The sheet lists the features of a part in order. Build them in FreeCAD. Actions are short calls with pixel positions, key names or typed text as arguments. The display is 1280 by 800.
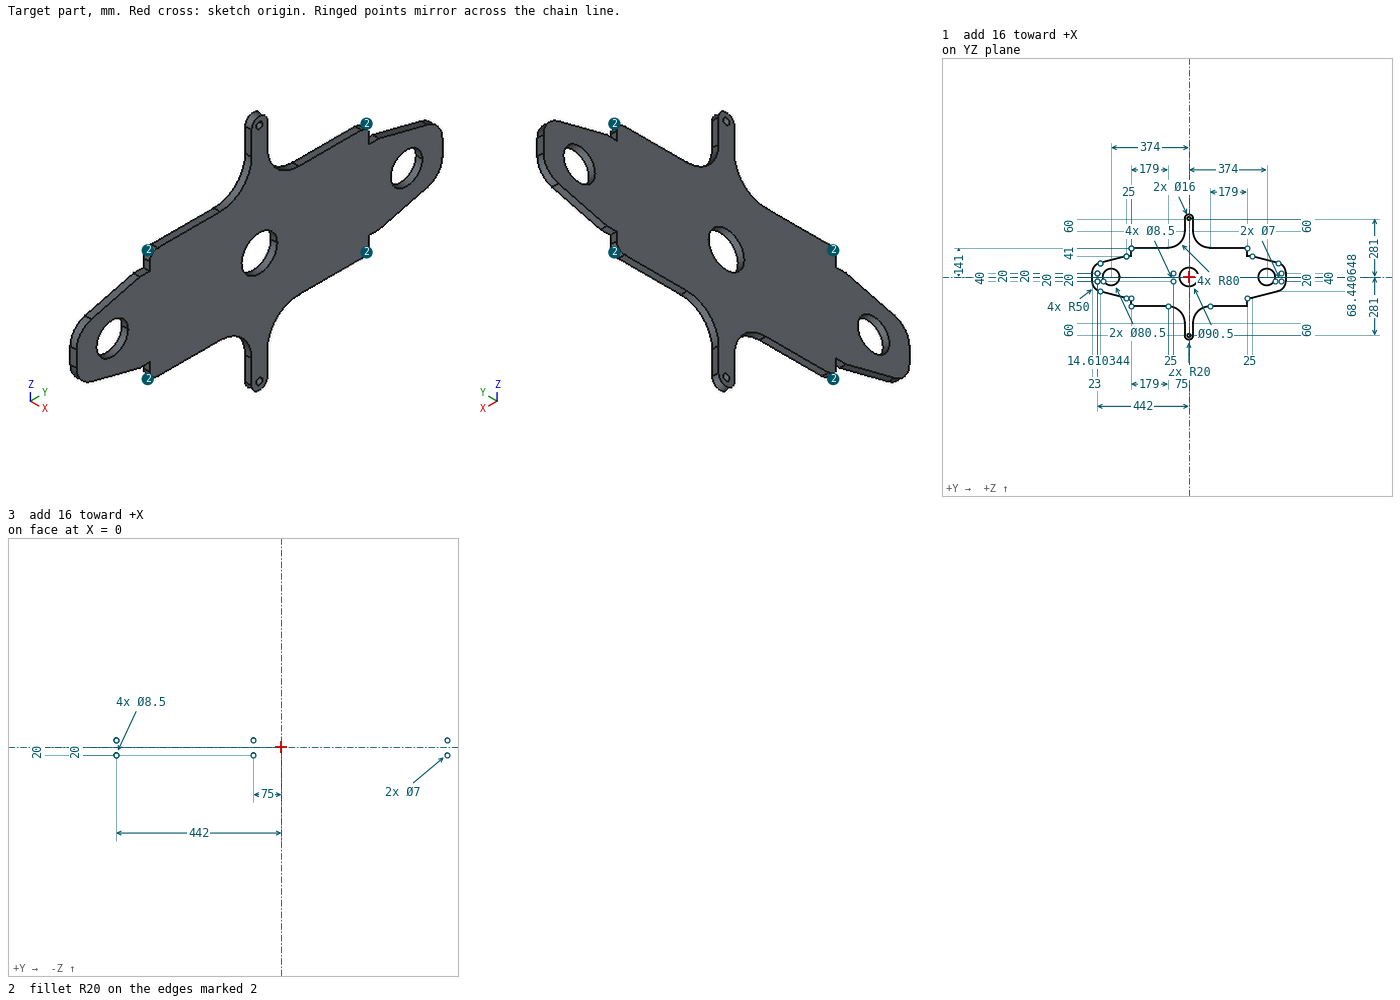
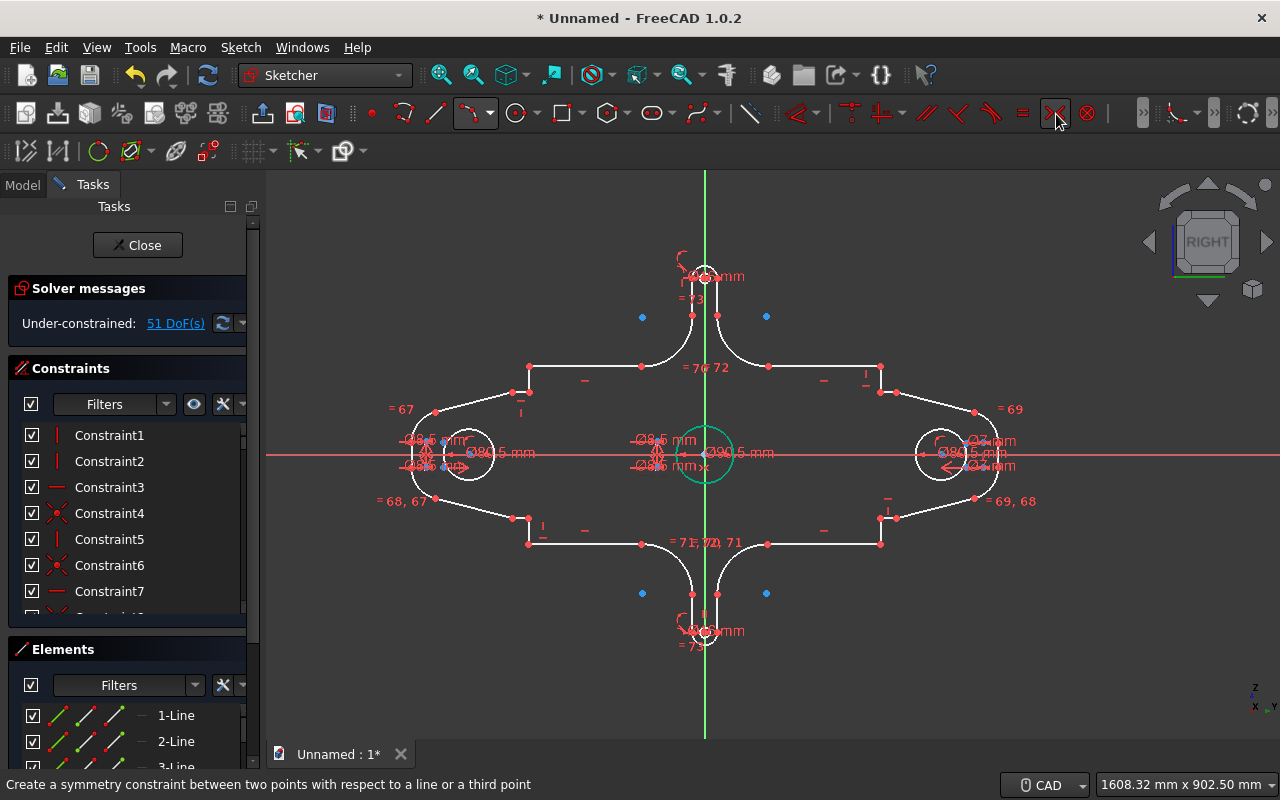
click(426, 468)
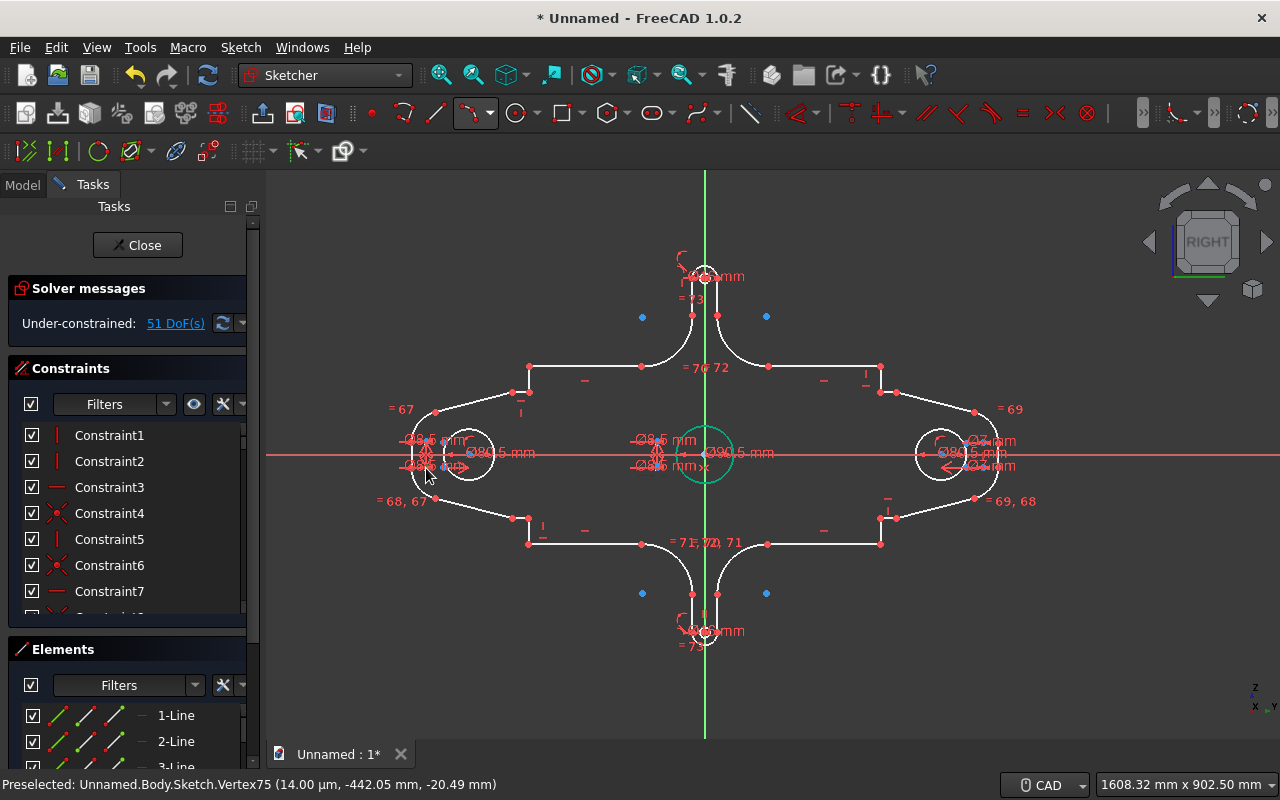
click(983, 468)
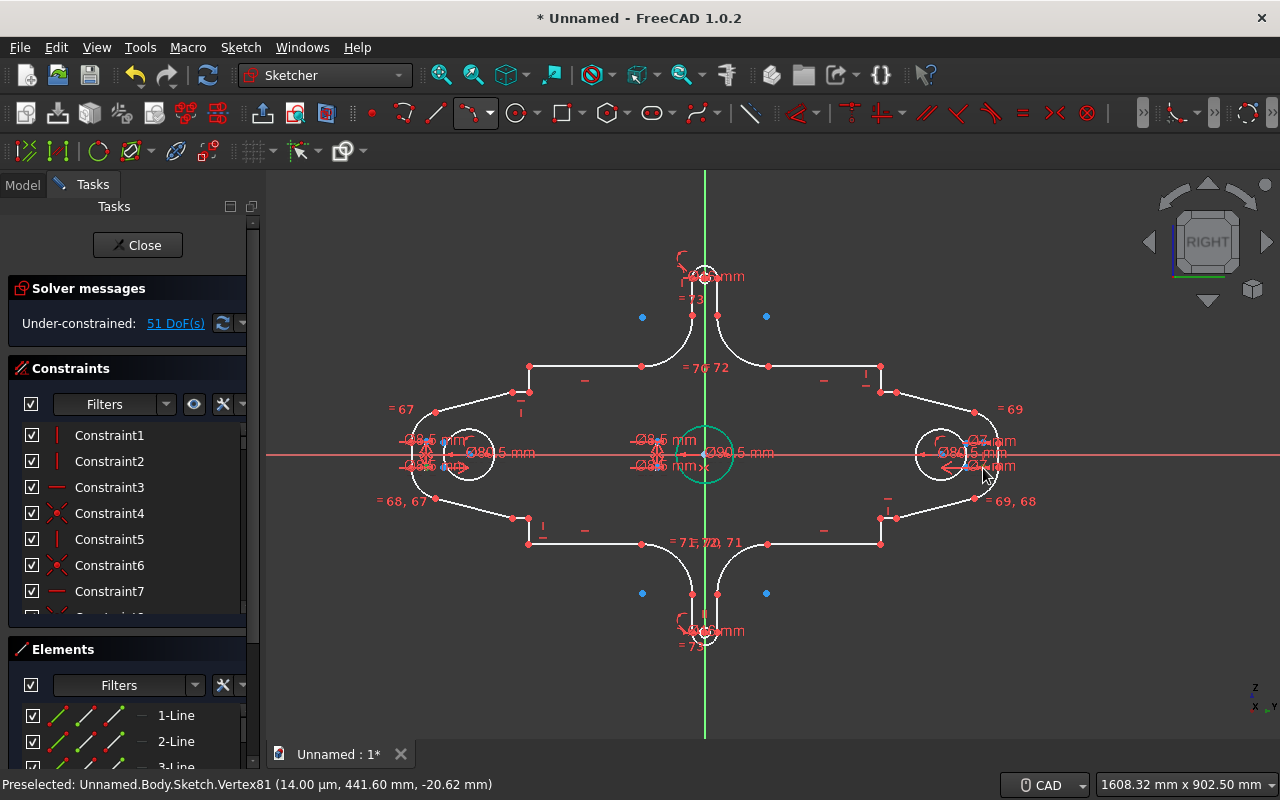
click(705, 528)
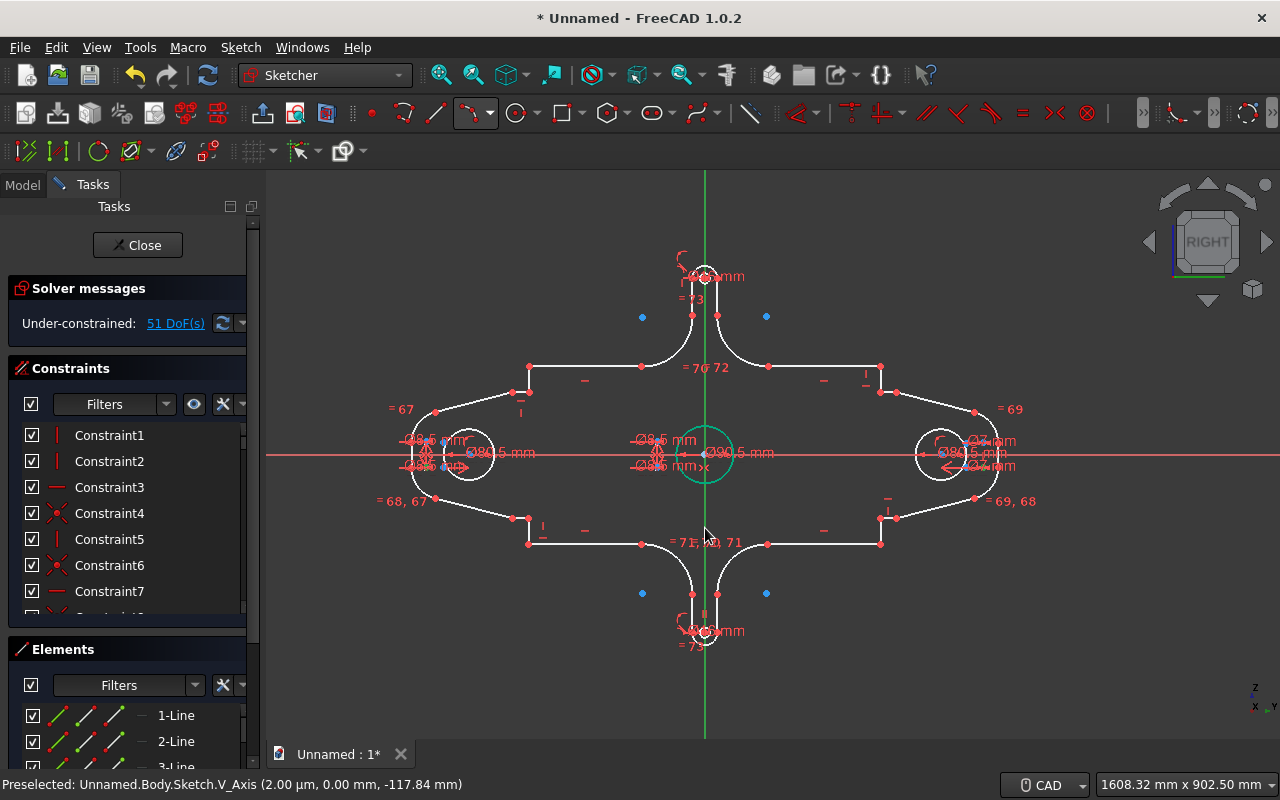
click(1056, 114)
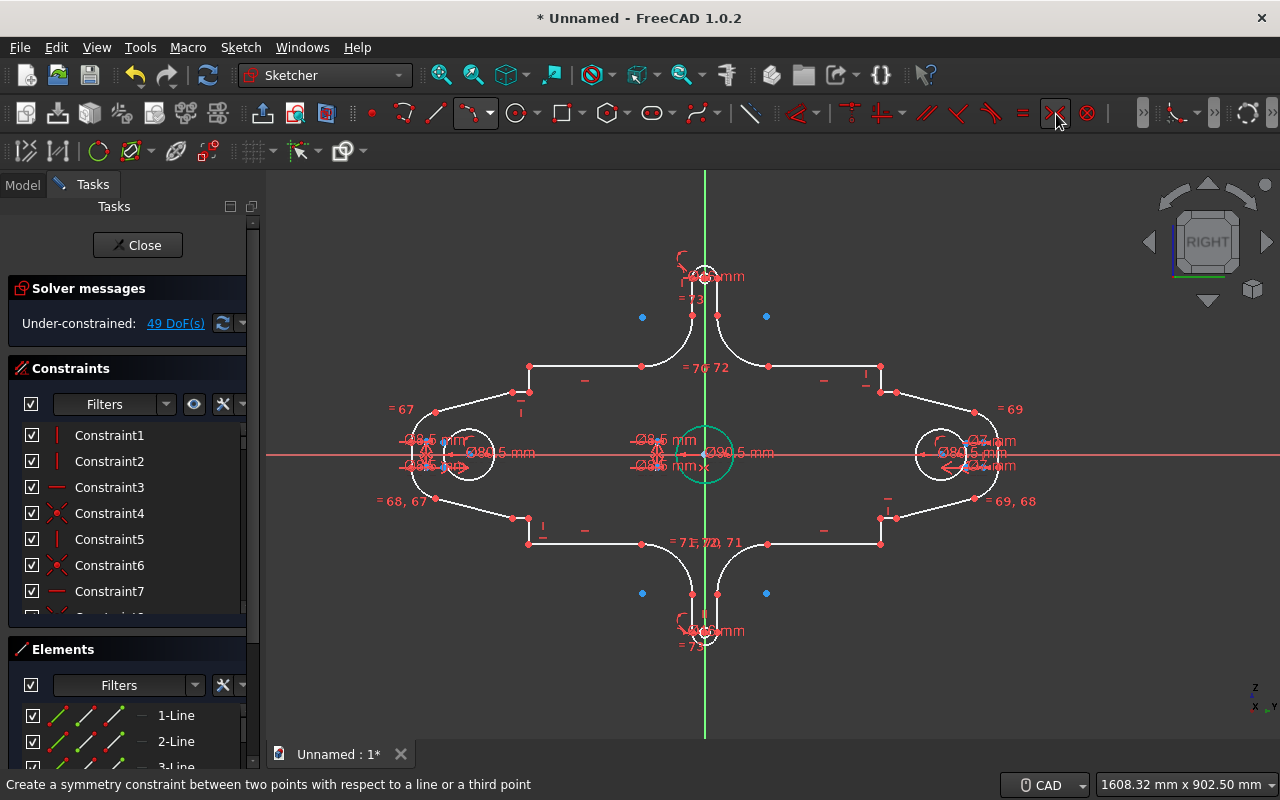
click(426, 442)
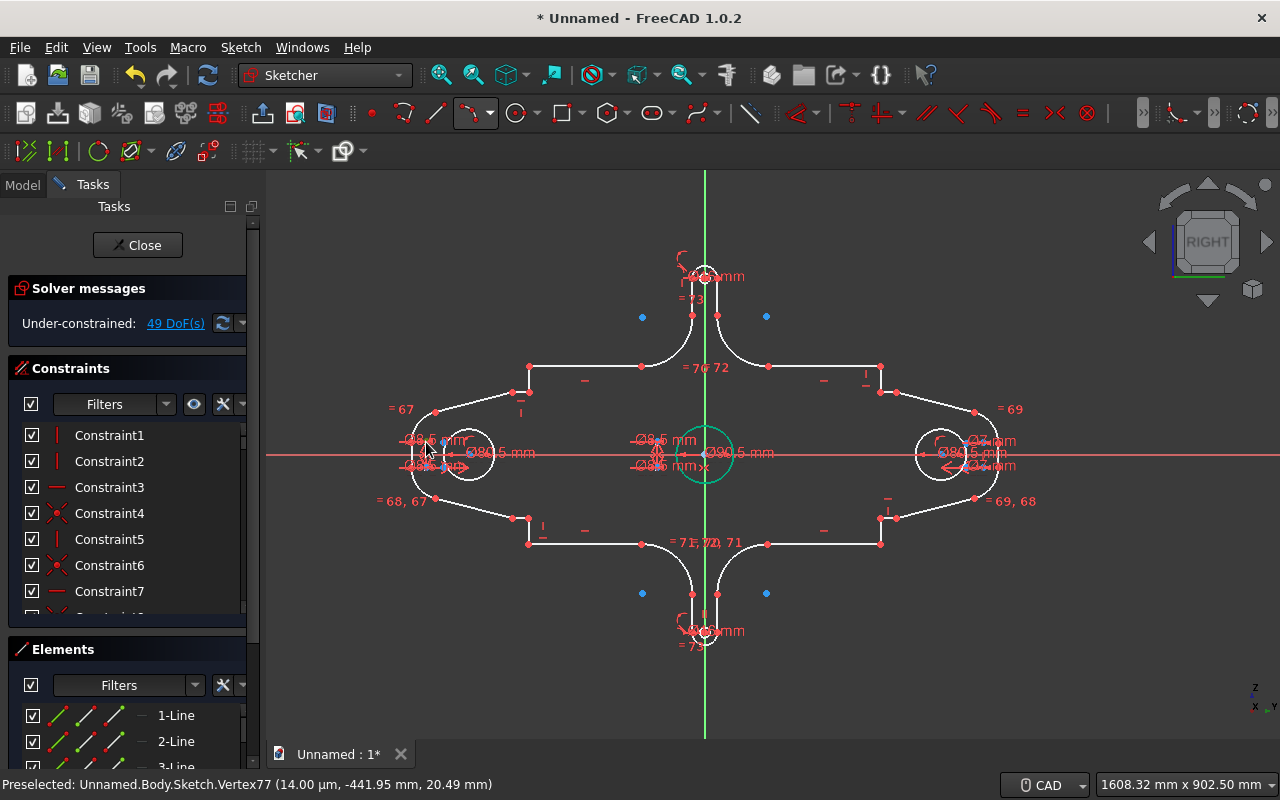
click(984, 443)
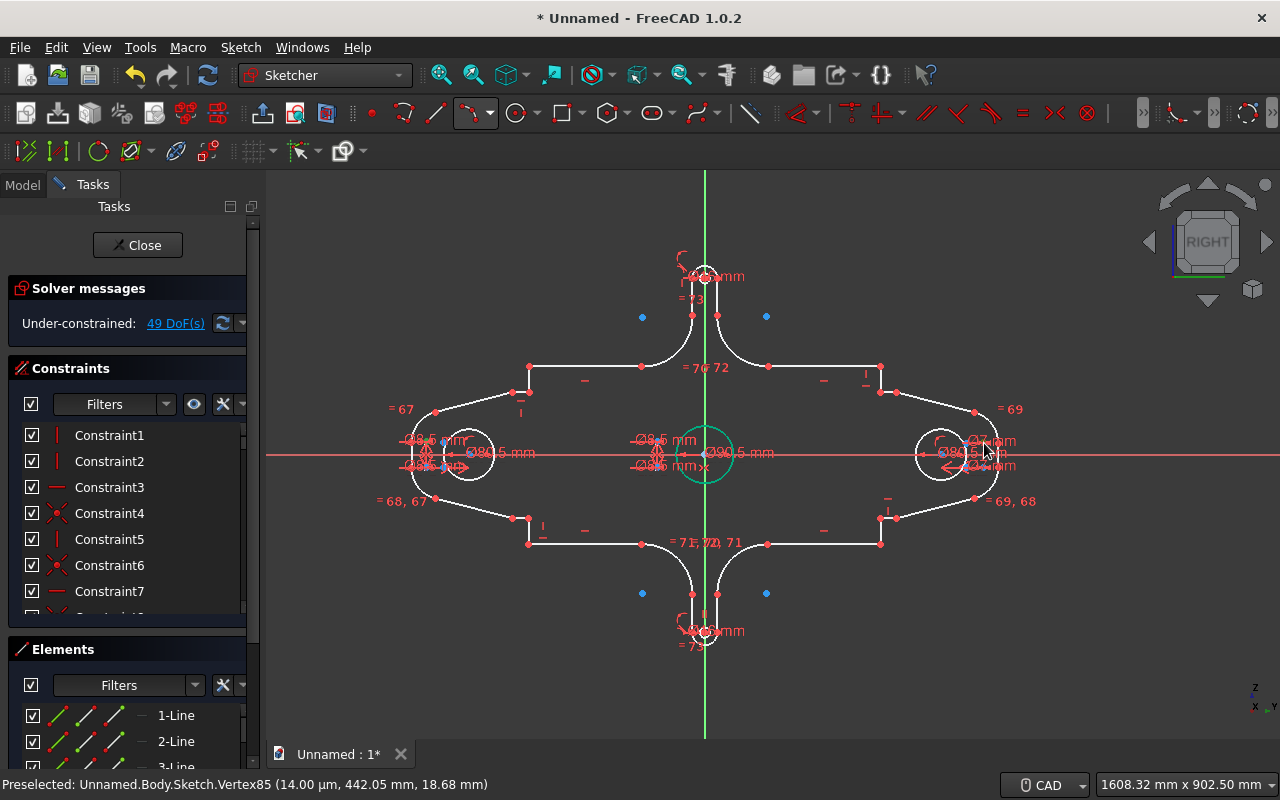
click(705, 528)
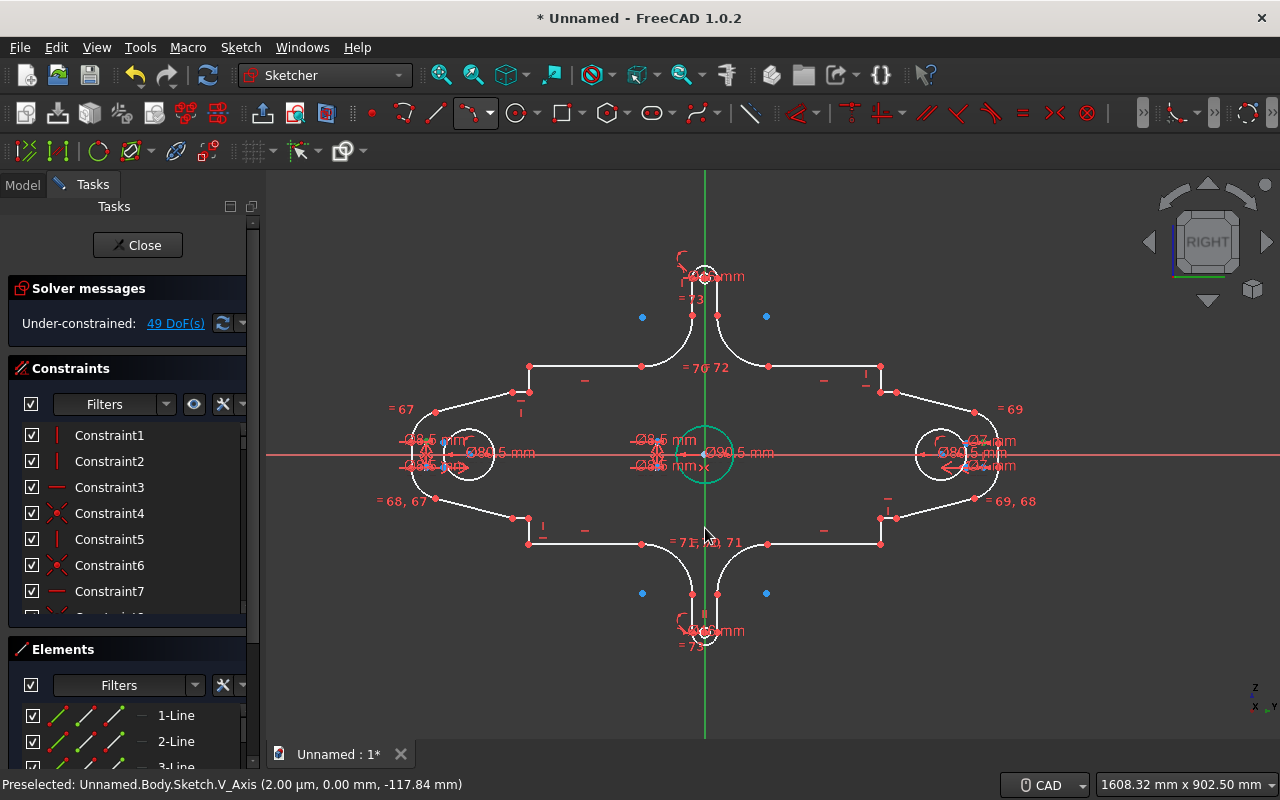
click(1056, 114)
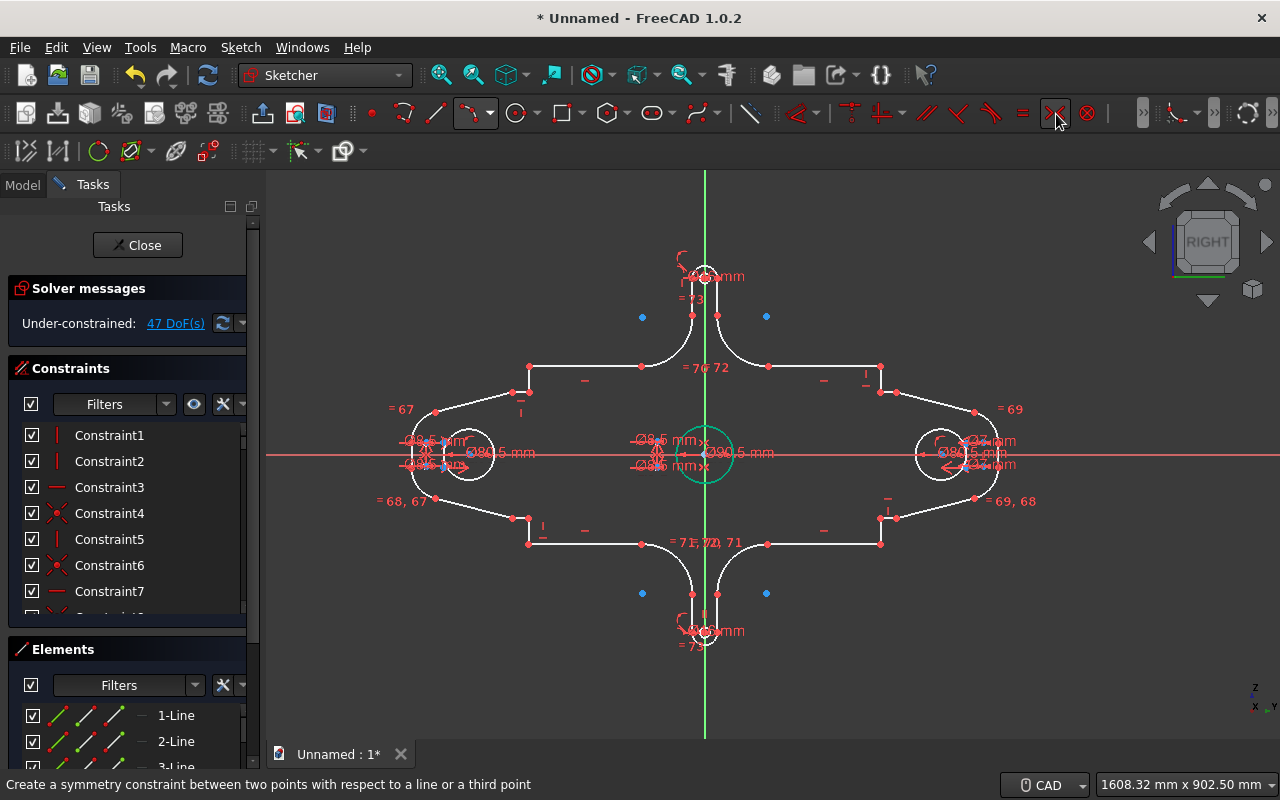
click(436, 412)